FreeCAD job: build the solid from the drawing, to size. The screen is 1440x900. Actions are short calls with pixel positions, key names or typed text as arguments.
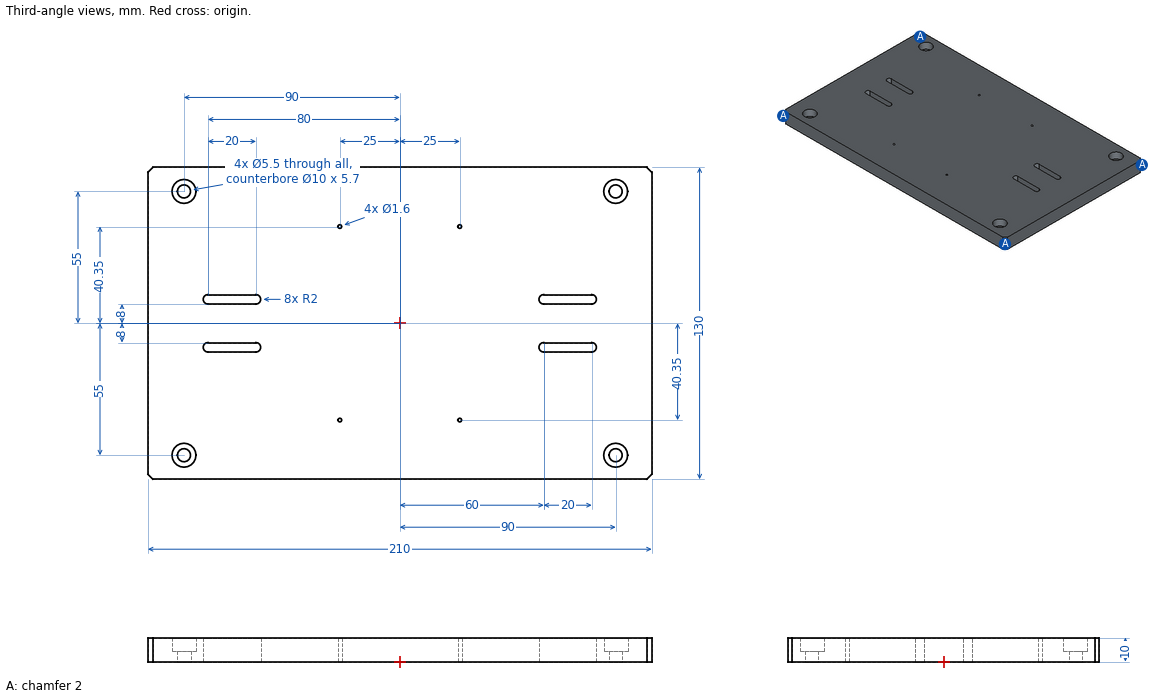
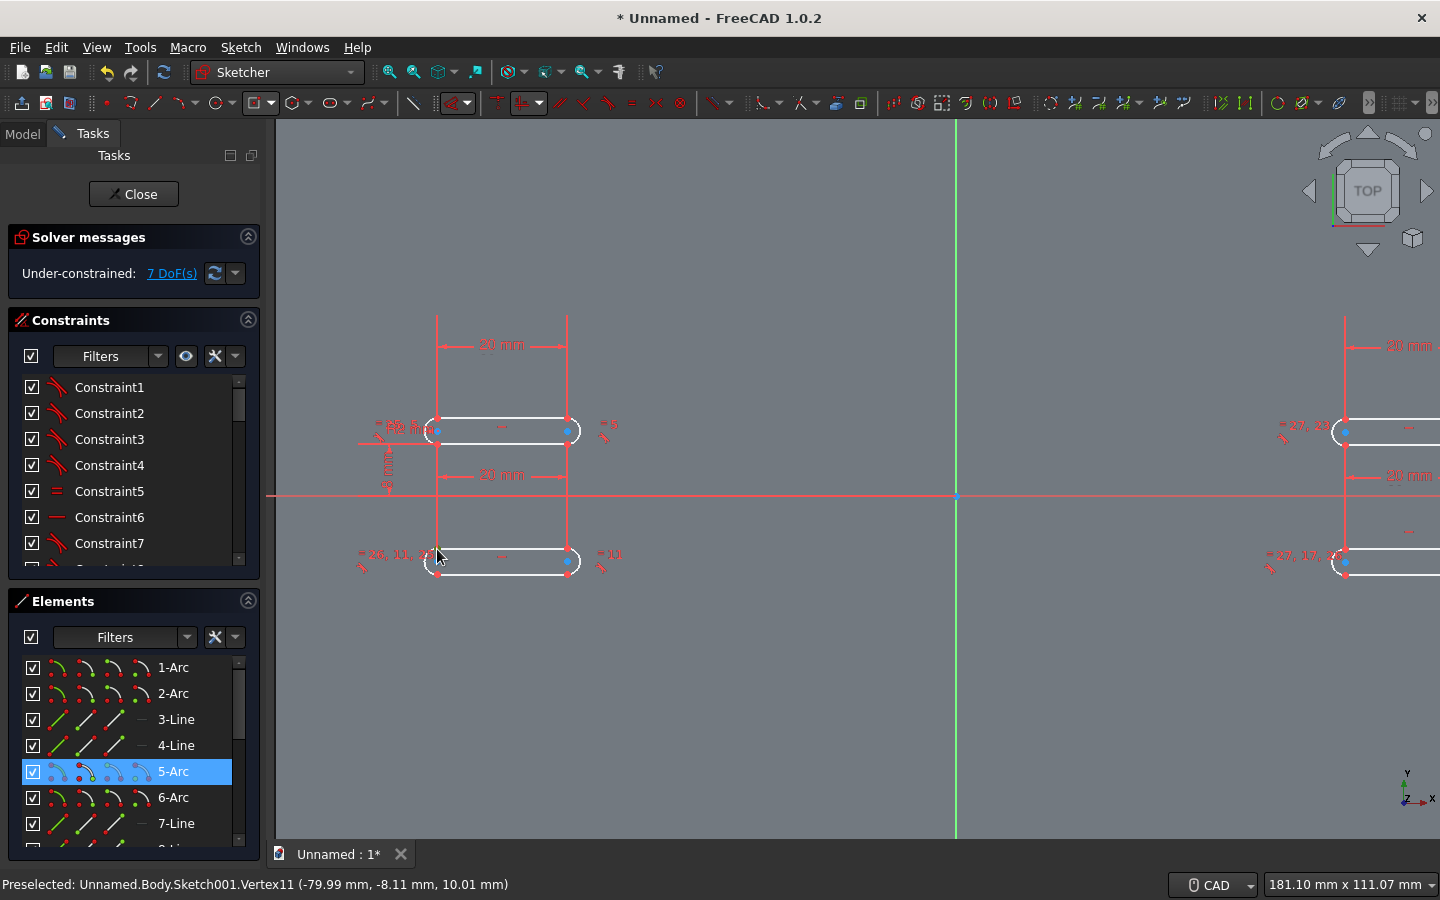
click(470, 104)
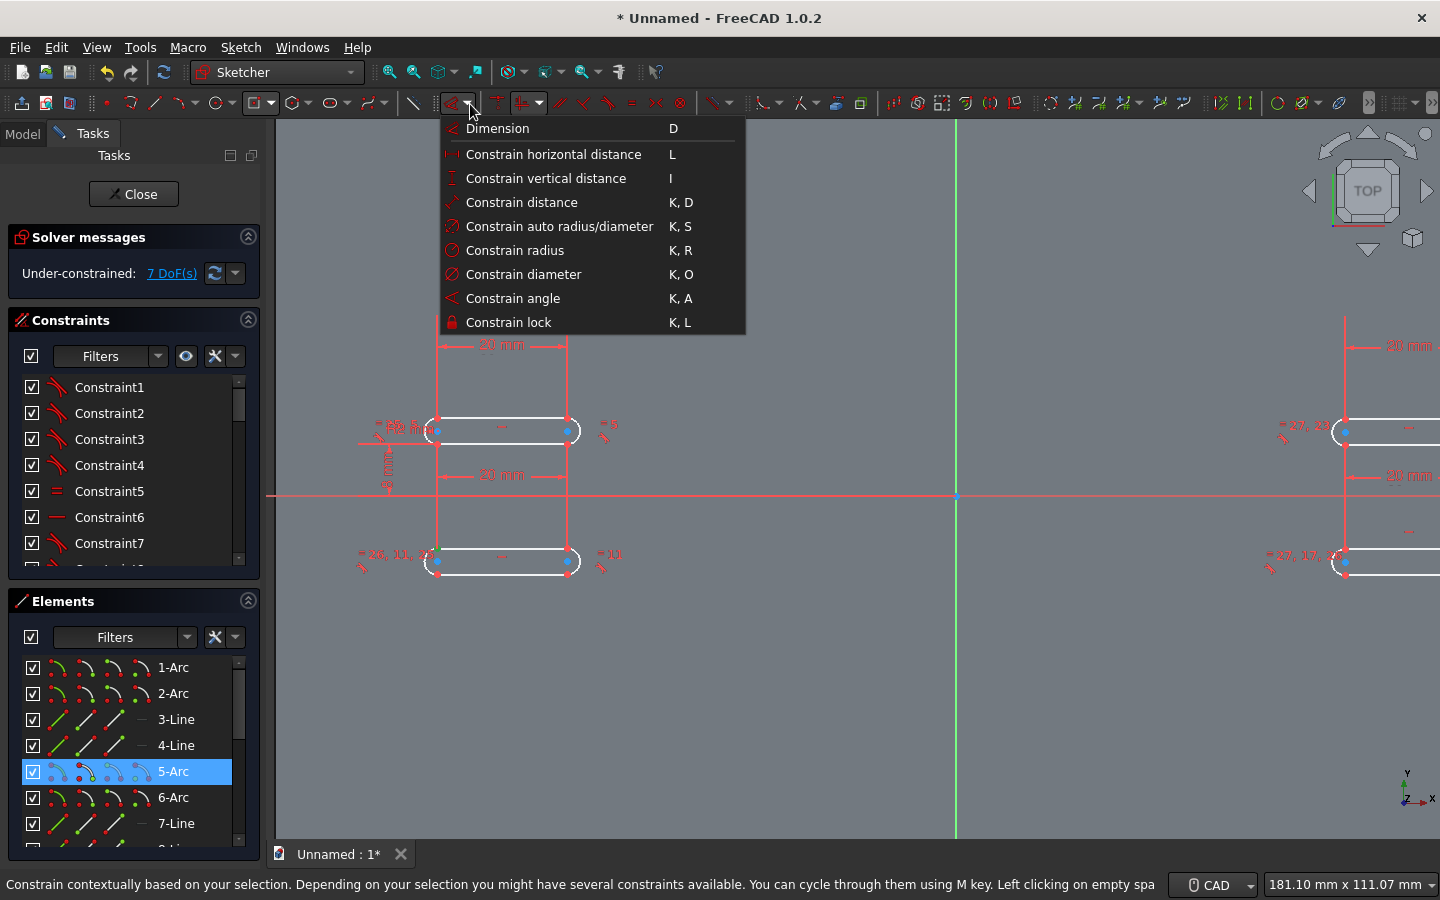
click(593, 178)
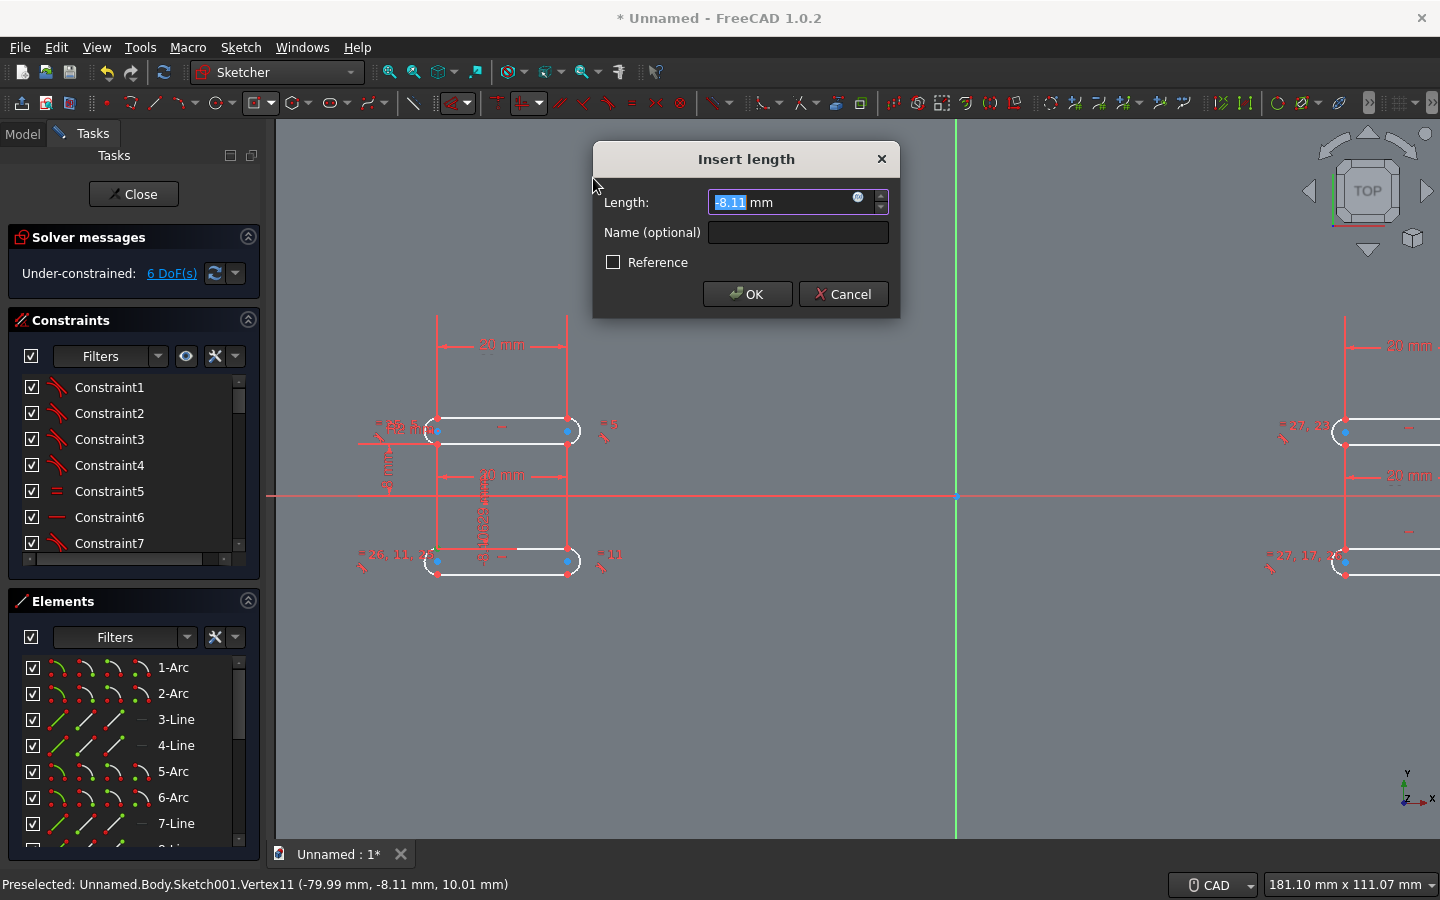
text(-8)
key(Return)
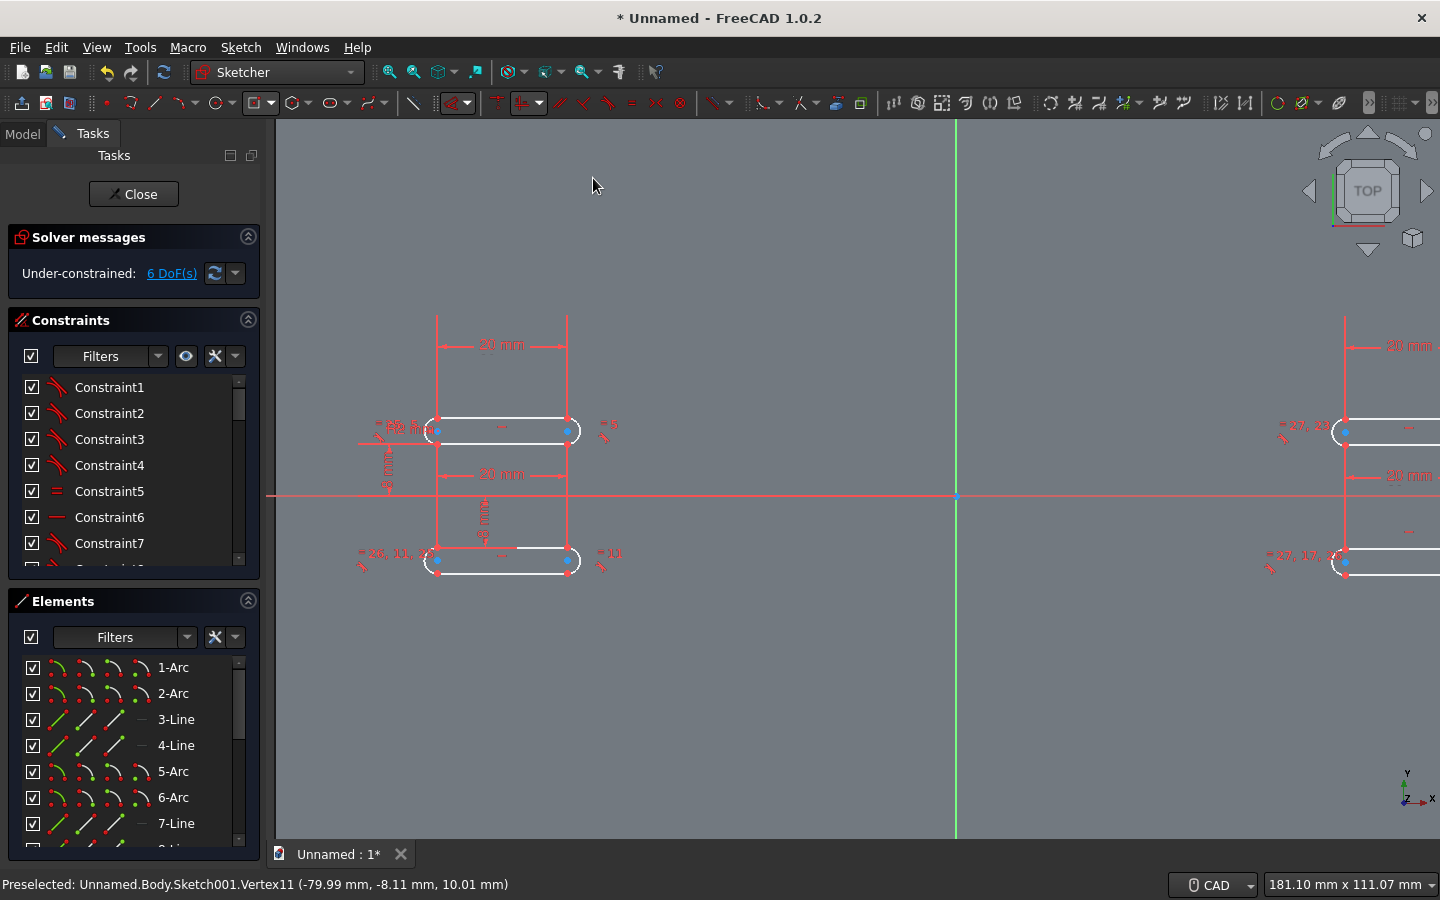
scroll(436, 444, down, 2)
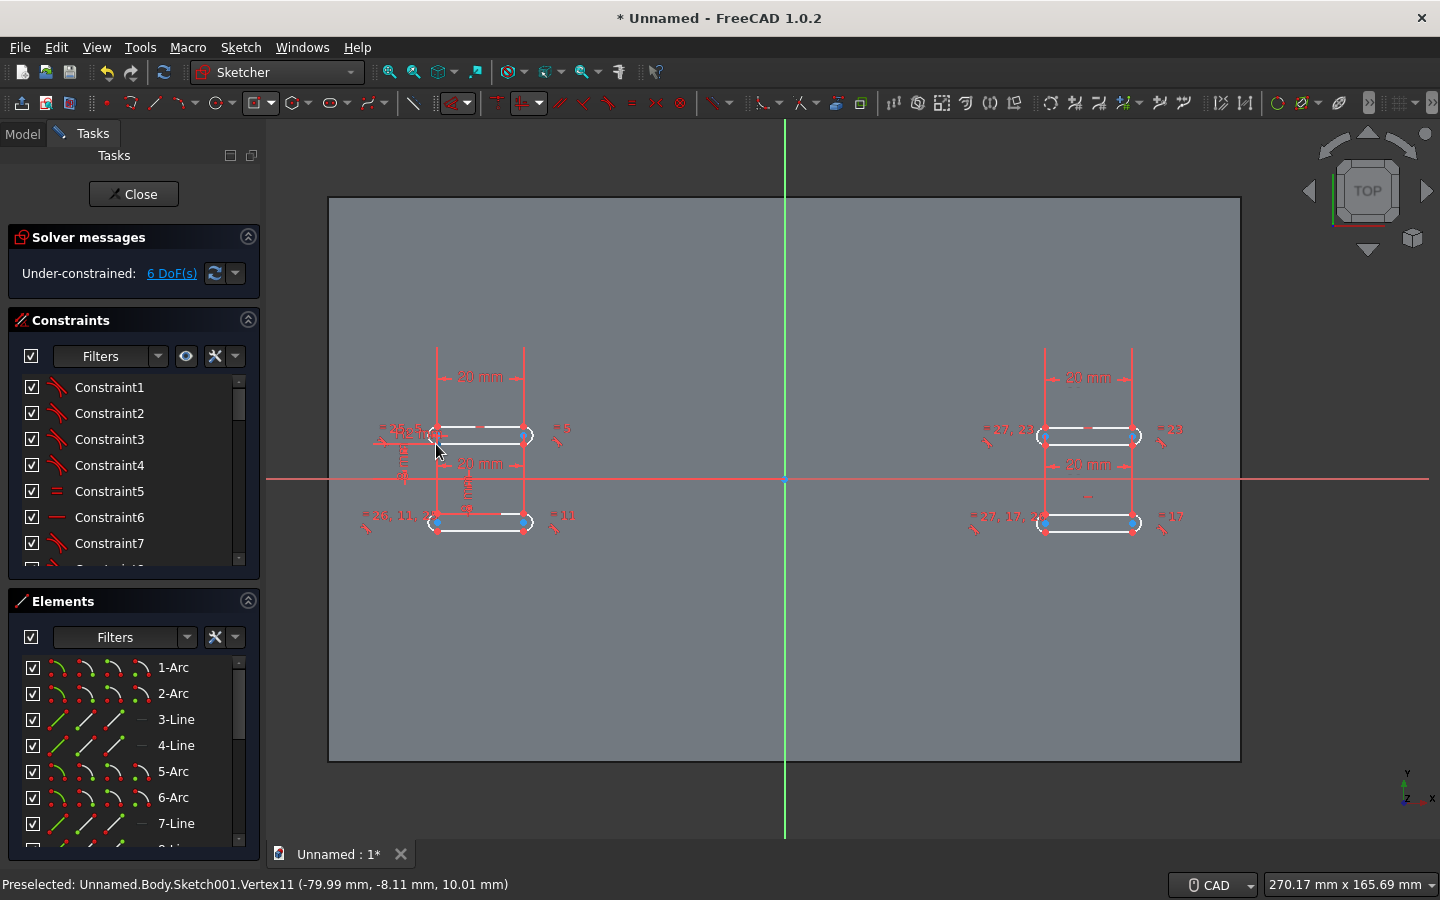
scroll(1045, 515, up, 2)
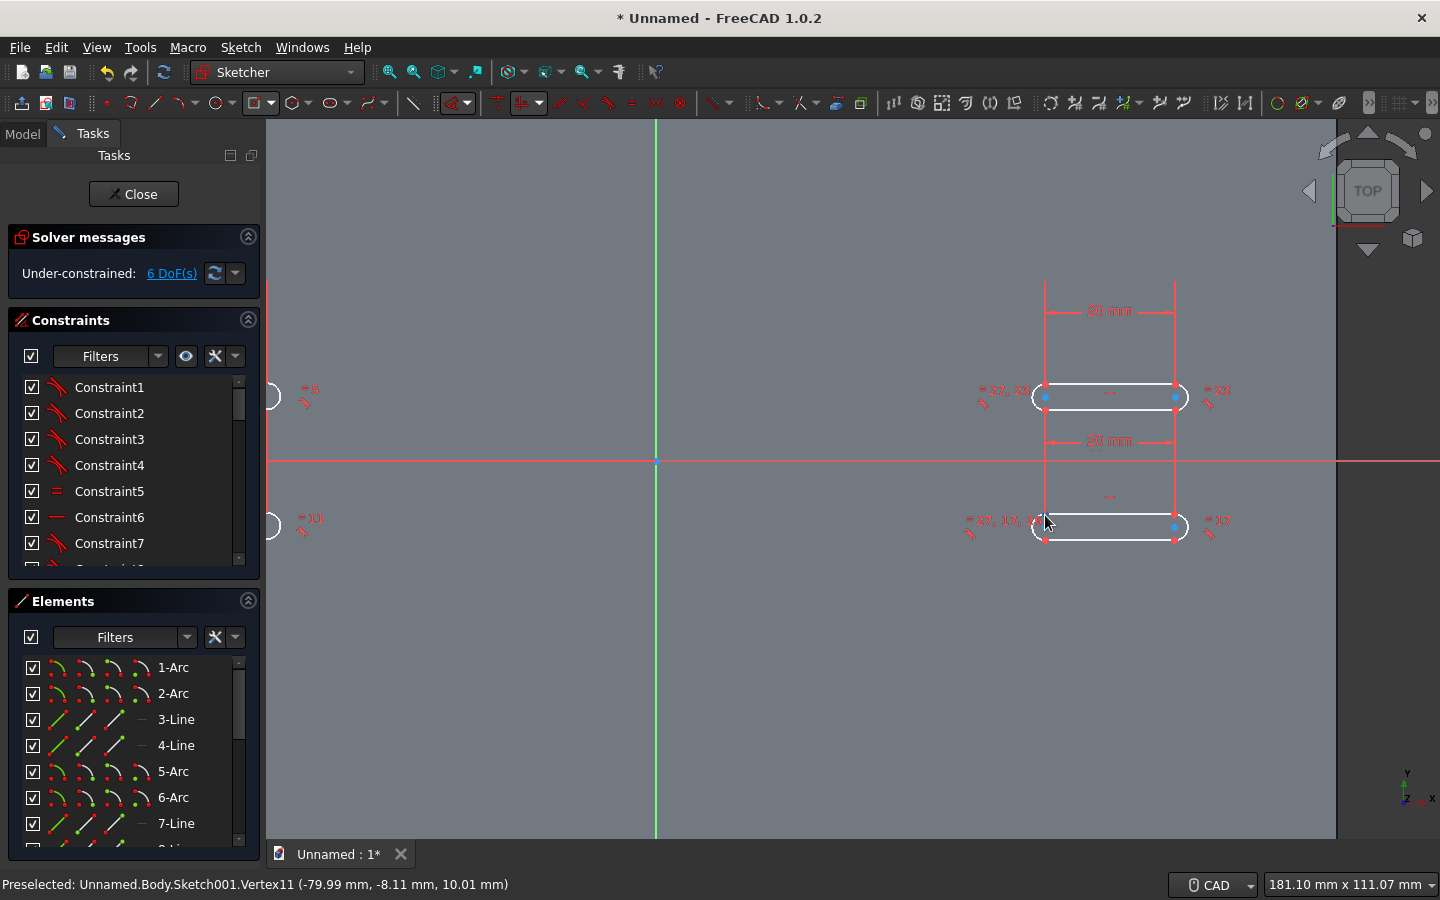
click(1045, 514)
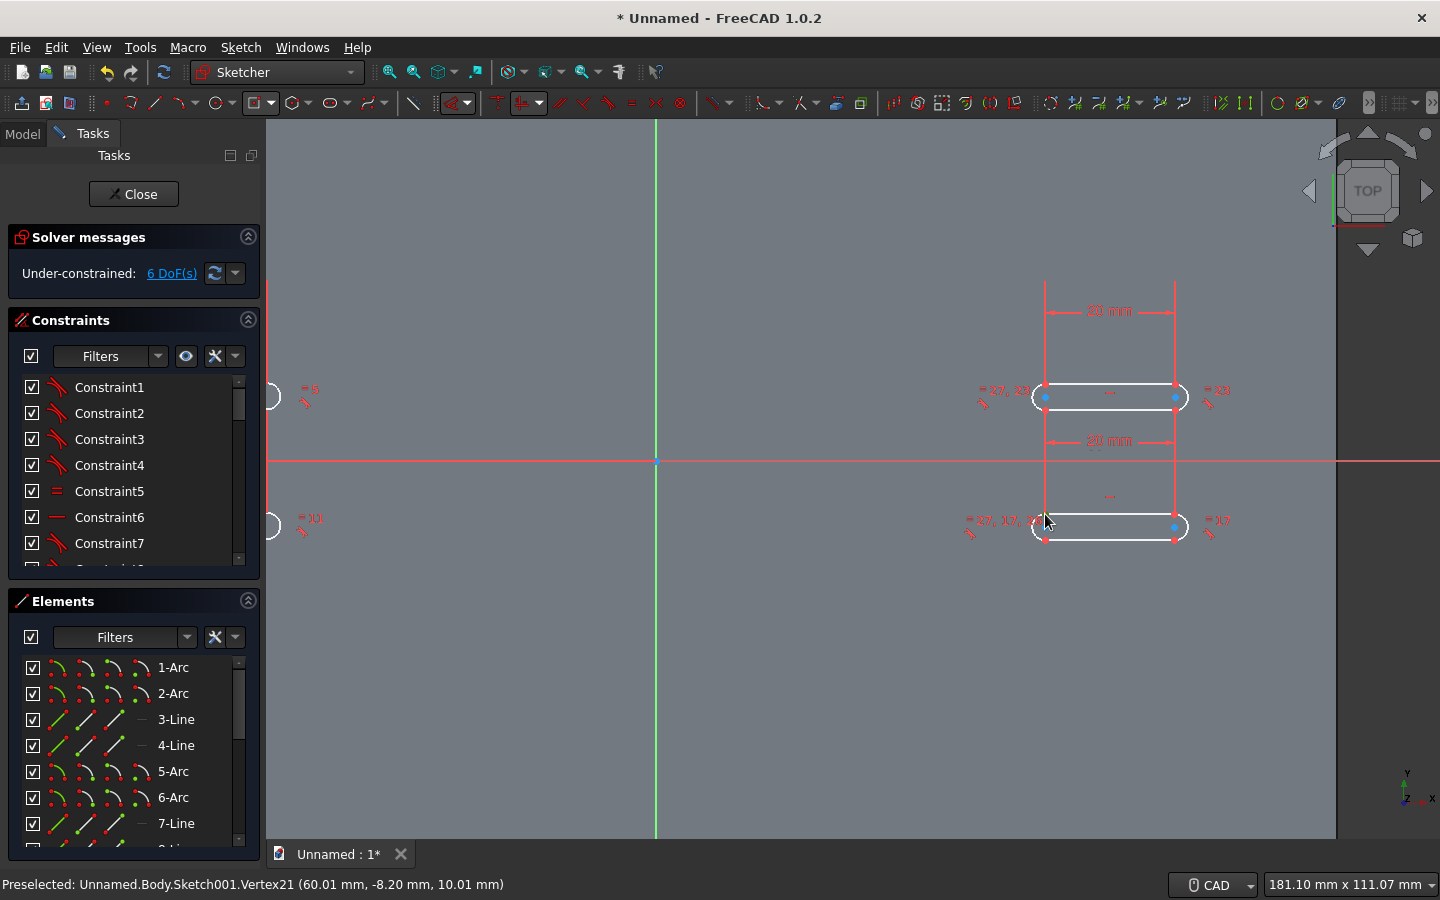
click(470, 104)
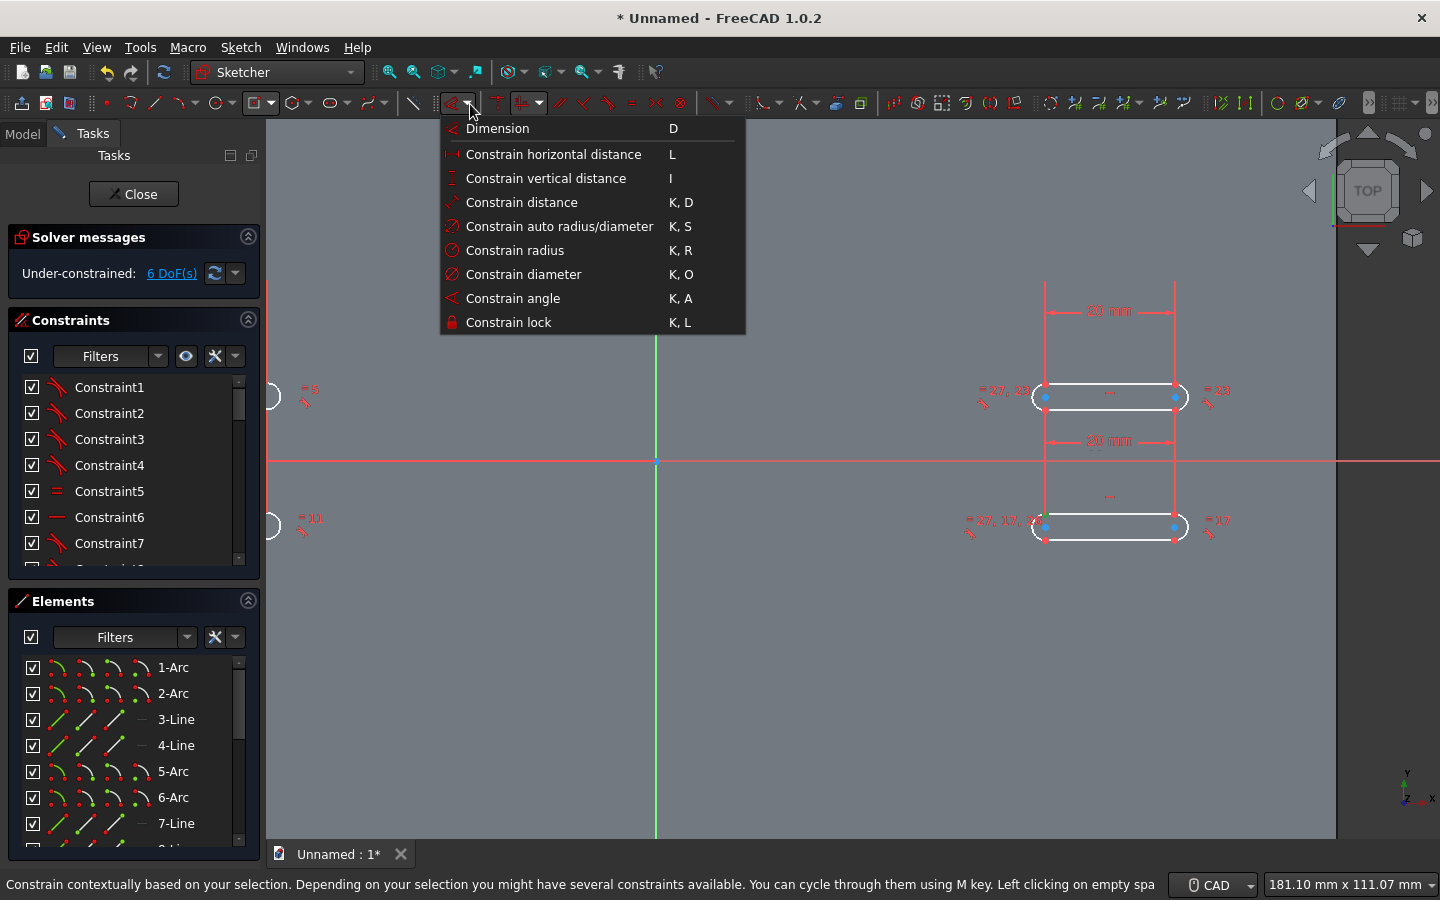
click(593, 178)